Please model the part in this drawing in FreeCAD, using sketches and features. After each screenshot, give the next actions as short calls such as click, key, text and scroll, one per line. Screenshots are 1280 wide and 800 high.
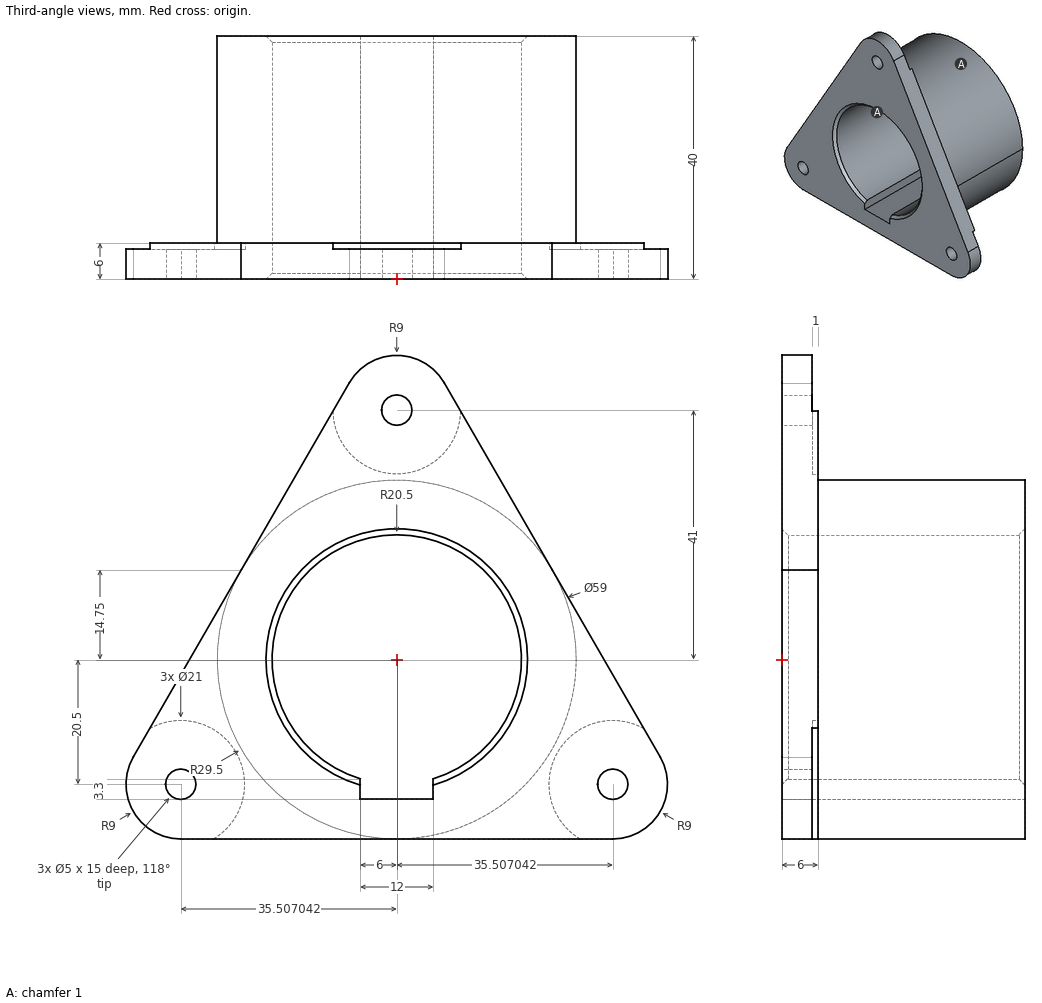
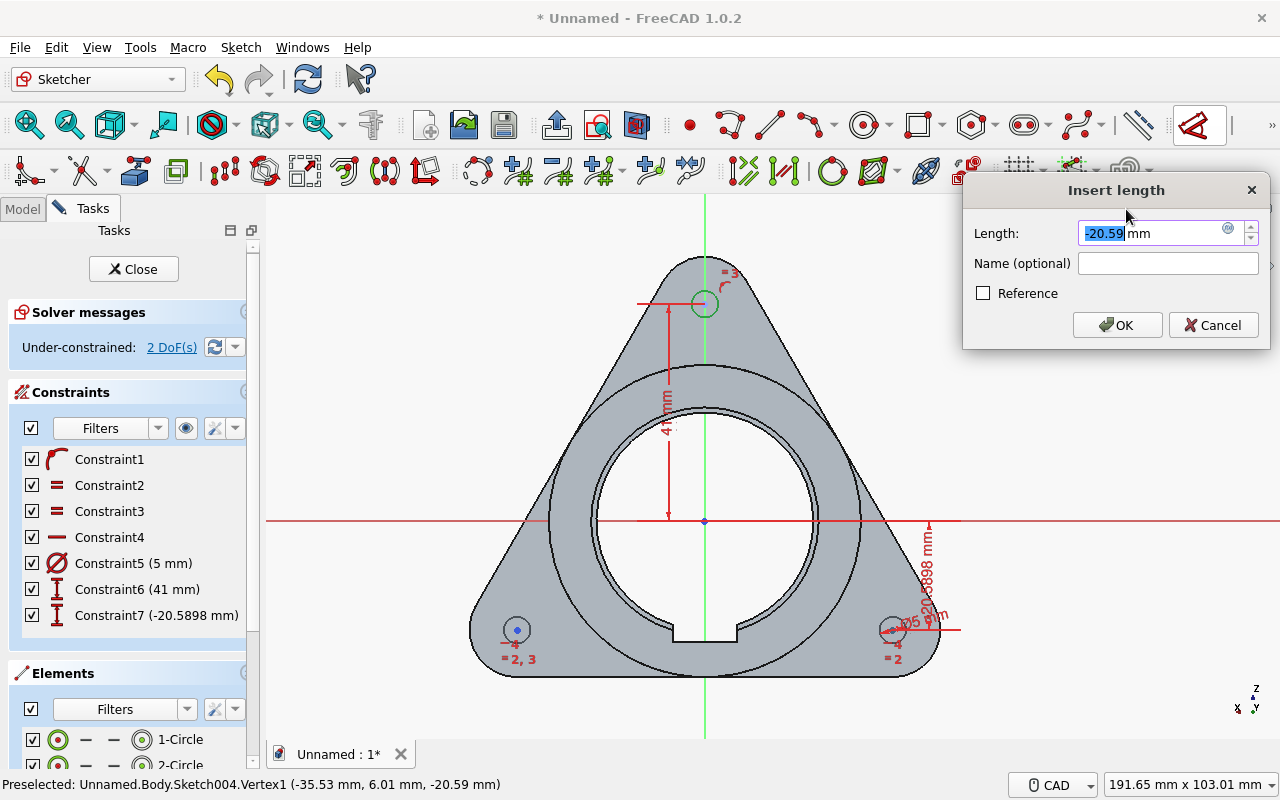
text(-20.5)
key(Return)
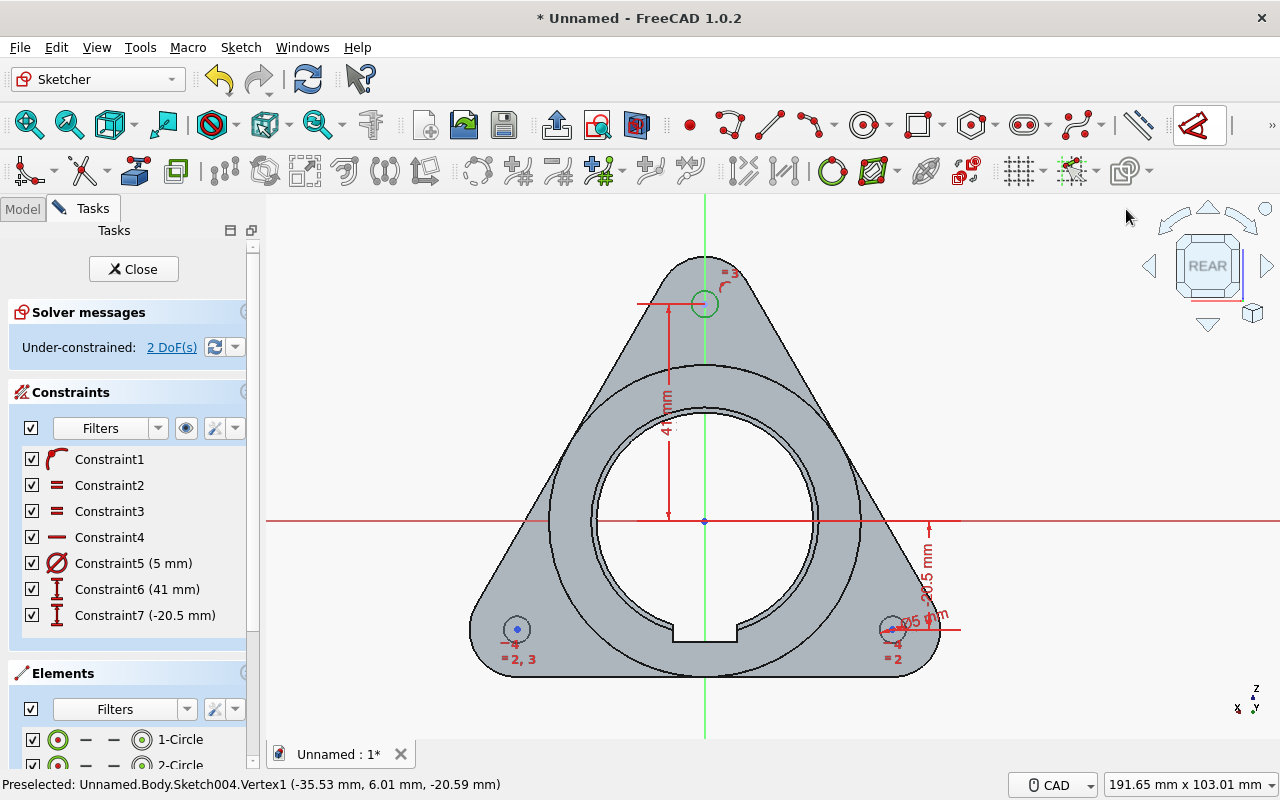
click(893, 630)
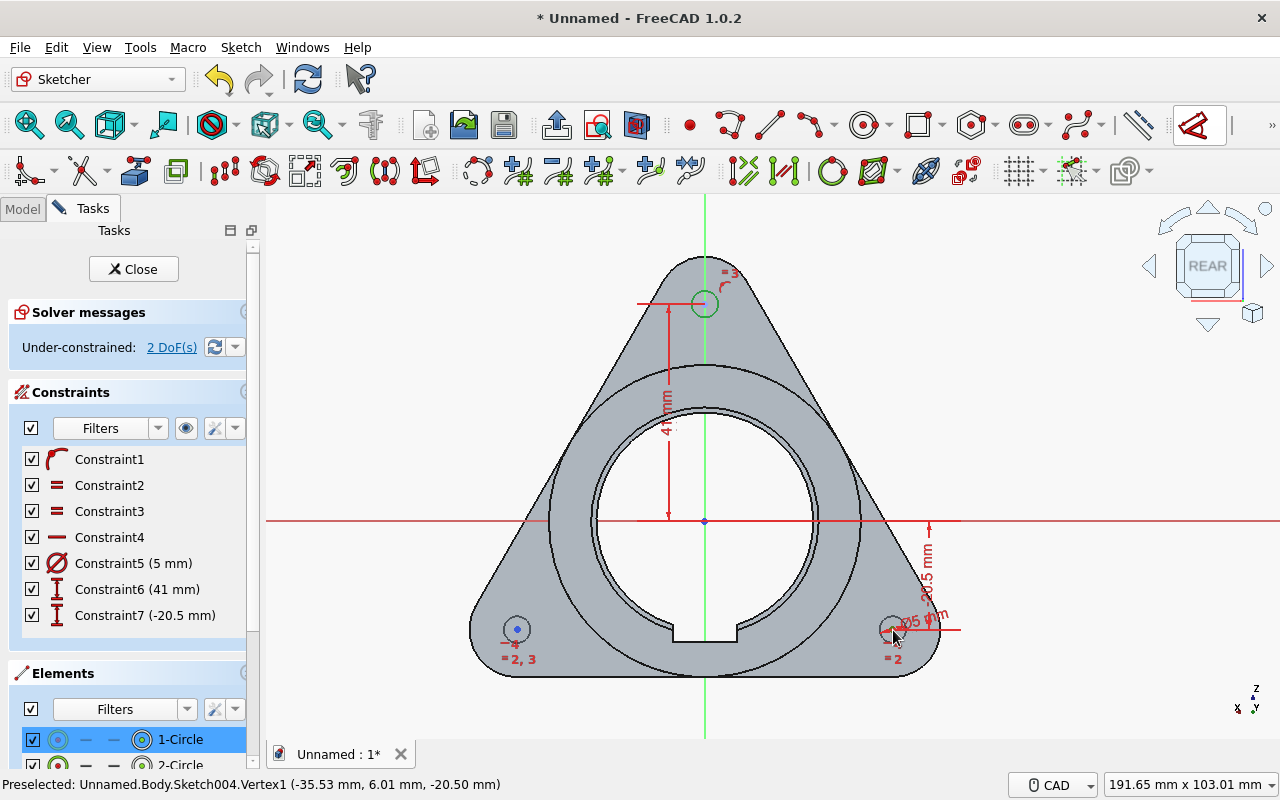
click(1220, 126)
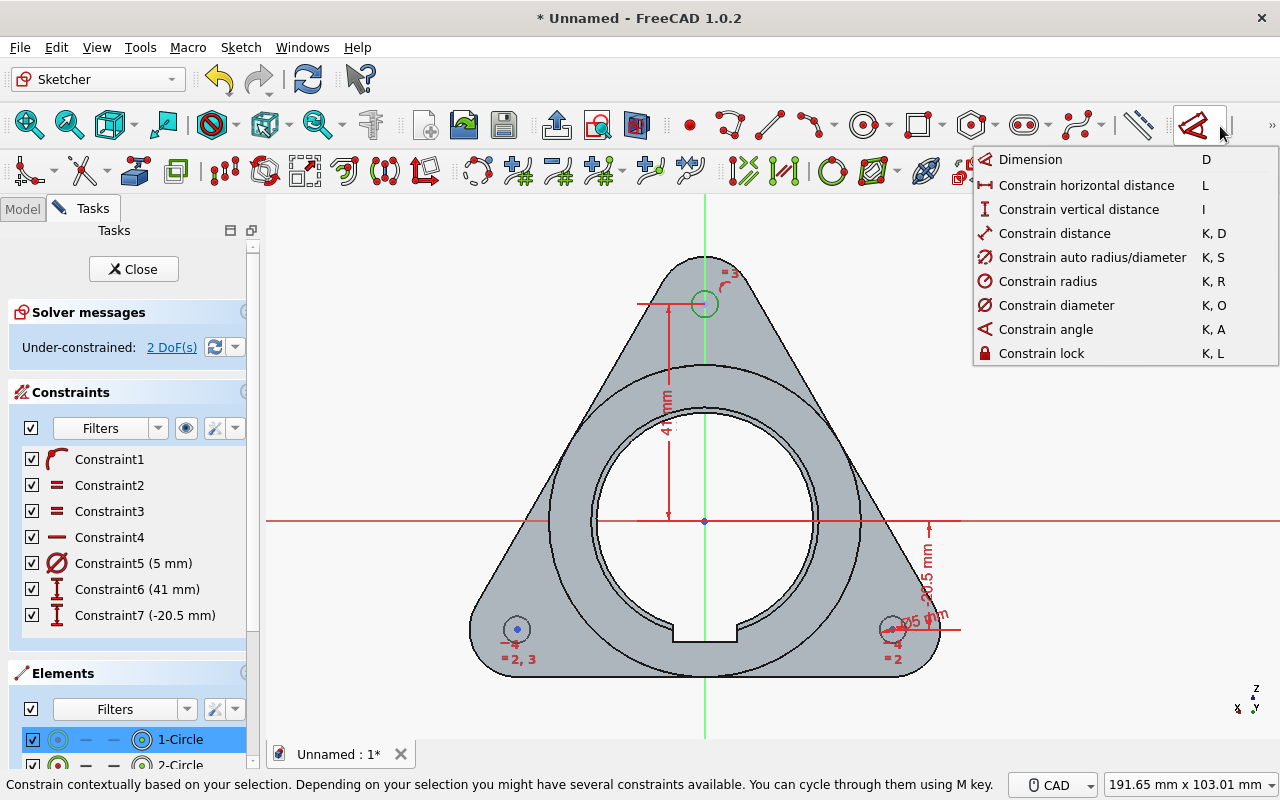
click(1126, 185)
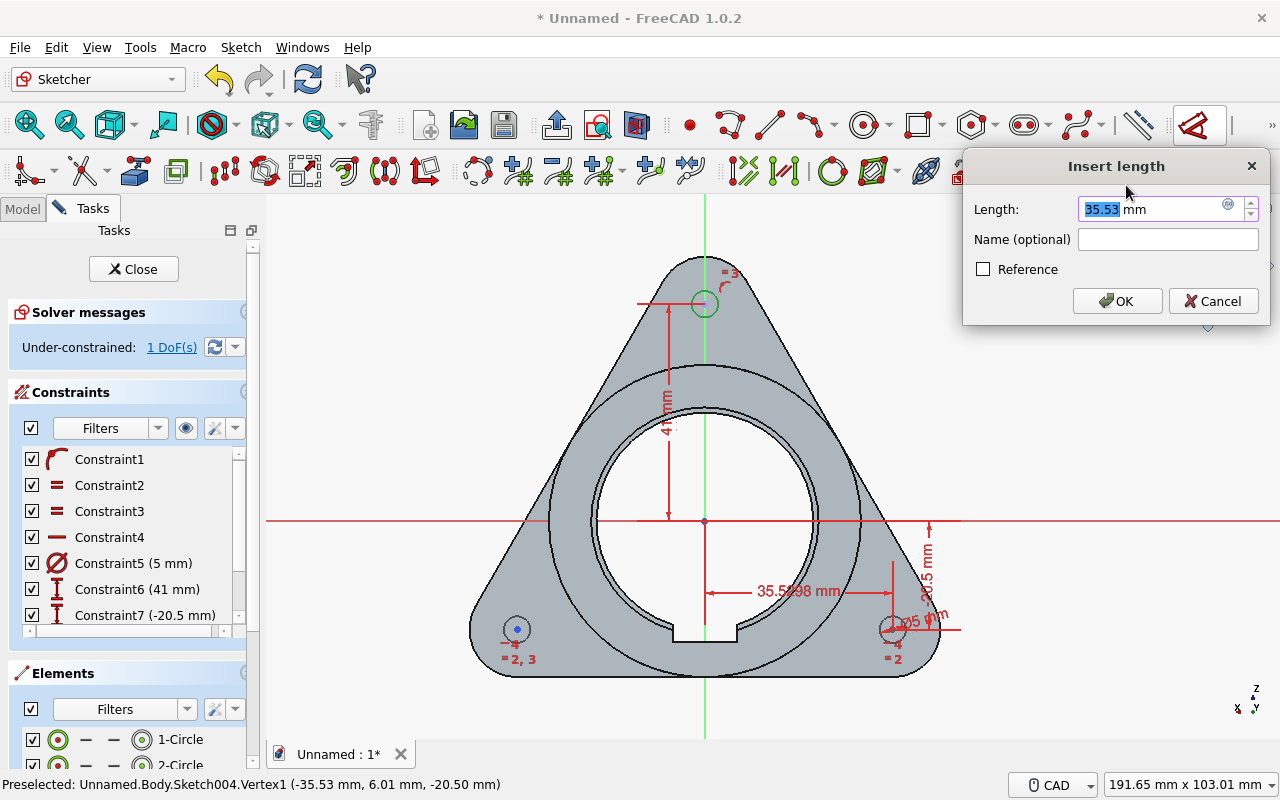
text(35.507042)
key(Return)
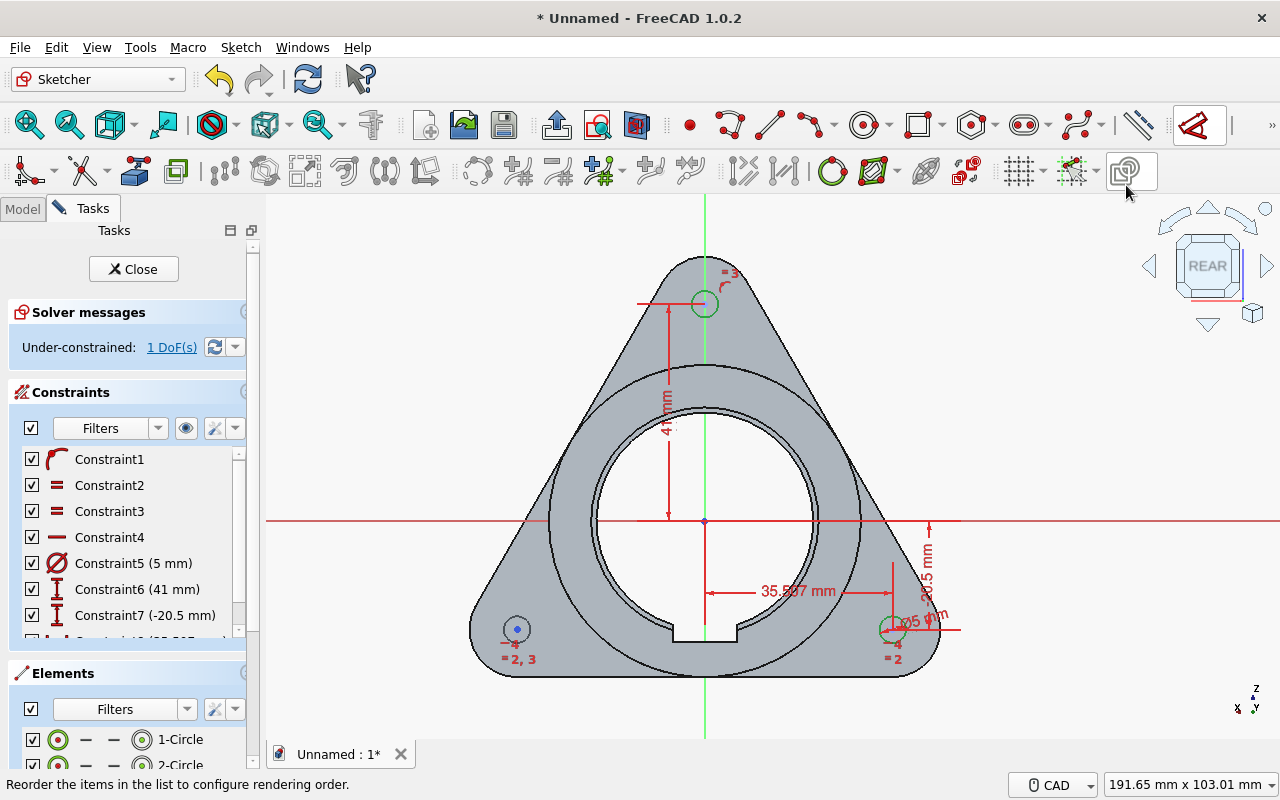
click(517, 630)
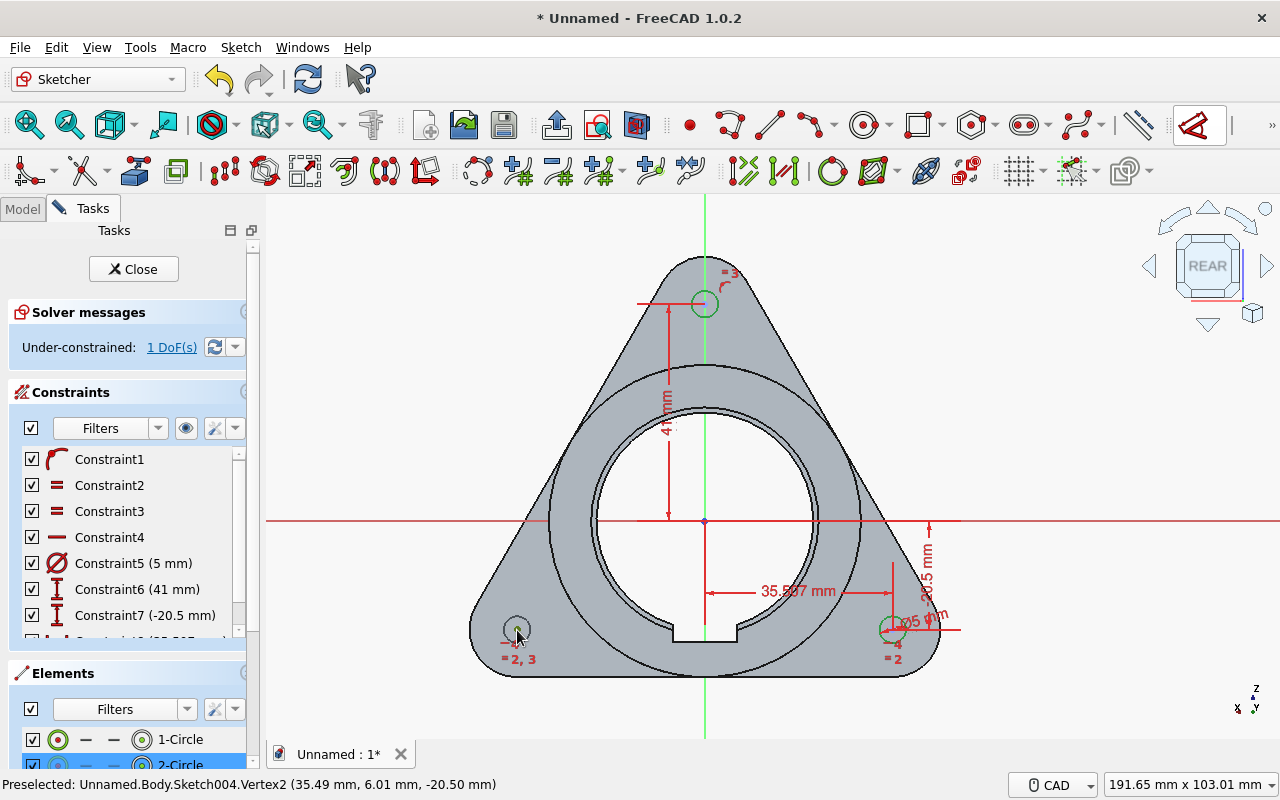
key(l)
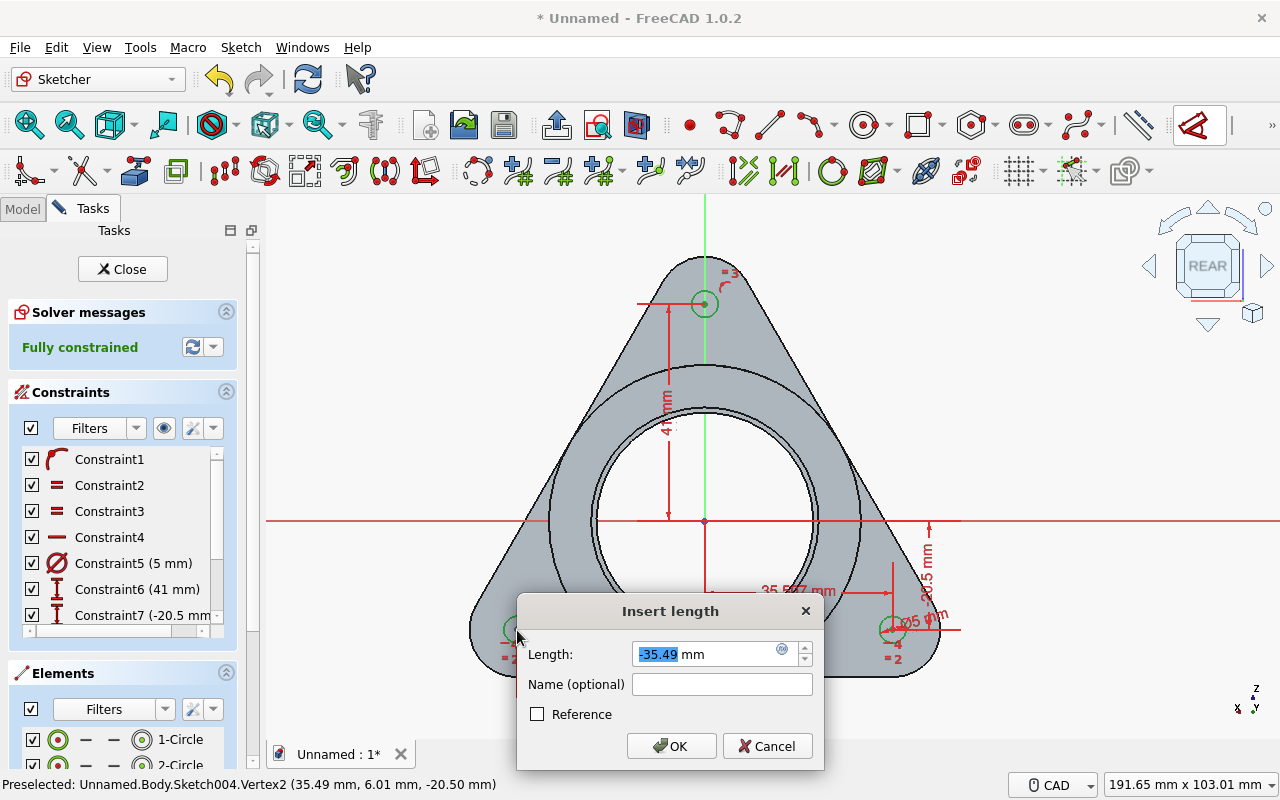
text(-35.507042)
key(Return)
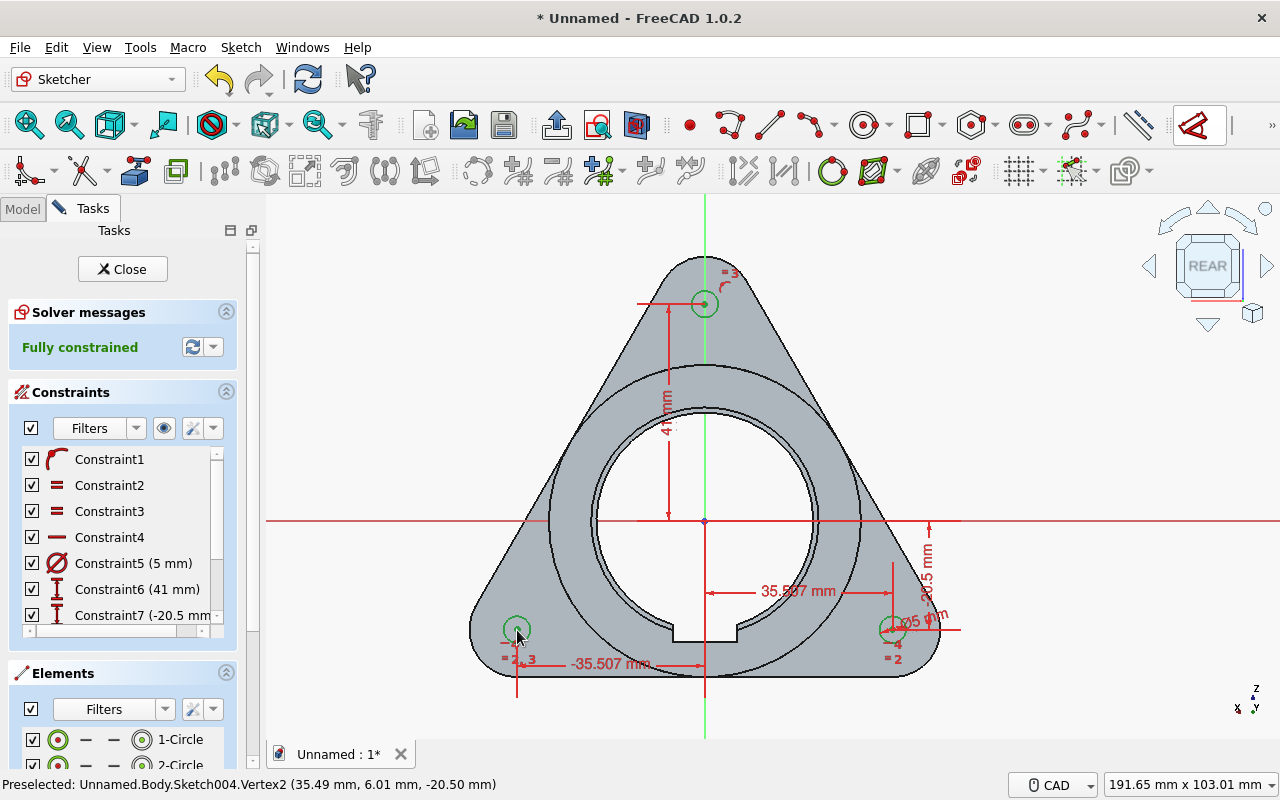
click(123, 269)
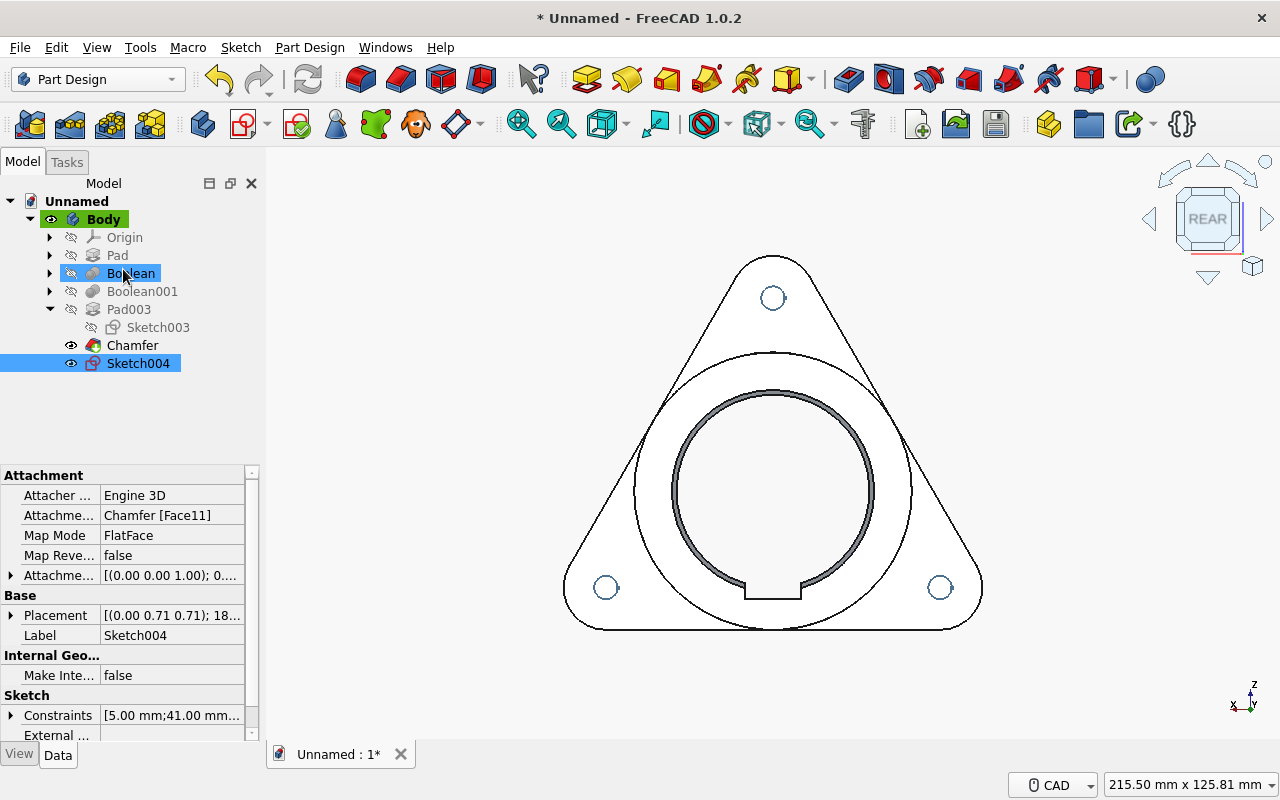
click(890, 80)